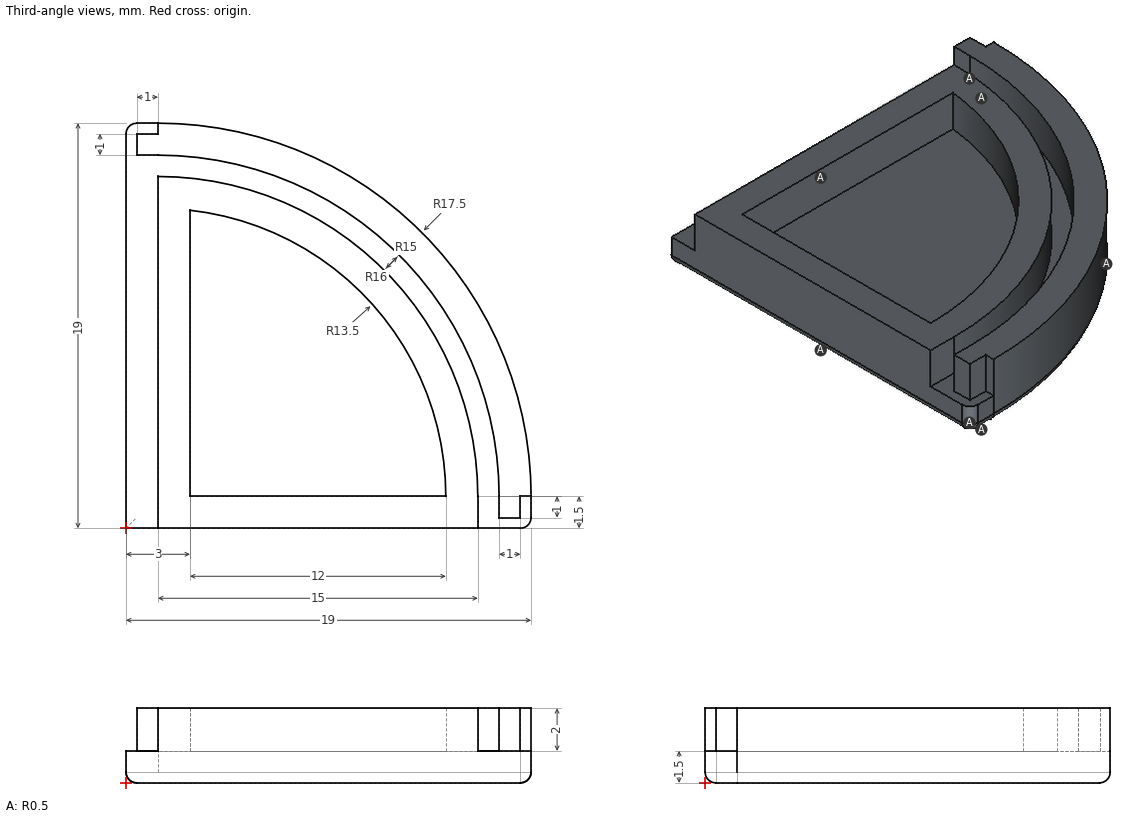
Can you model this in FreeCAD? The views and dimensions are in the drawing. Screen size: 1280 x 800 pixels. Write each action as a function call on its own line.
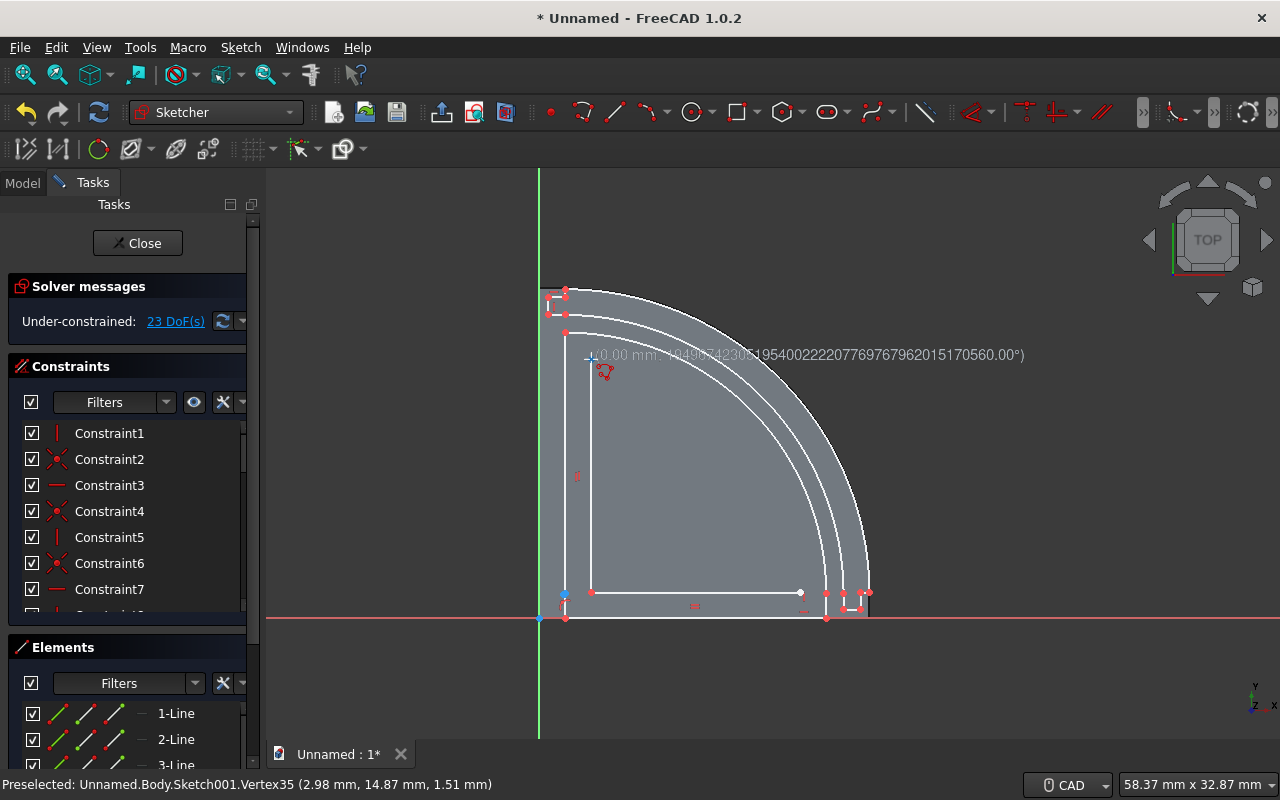
click(648, 112)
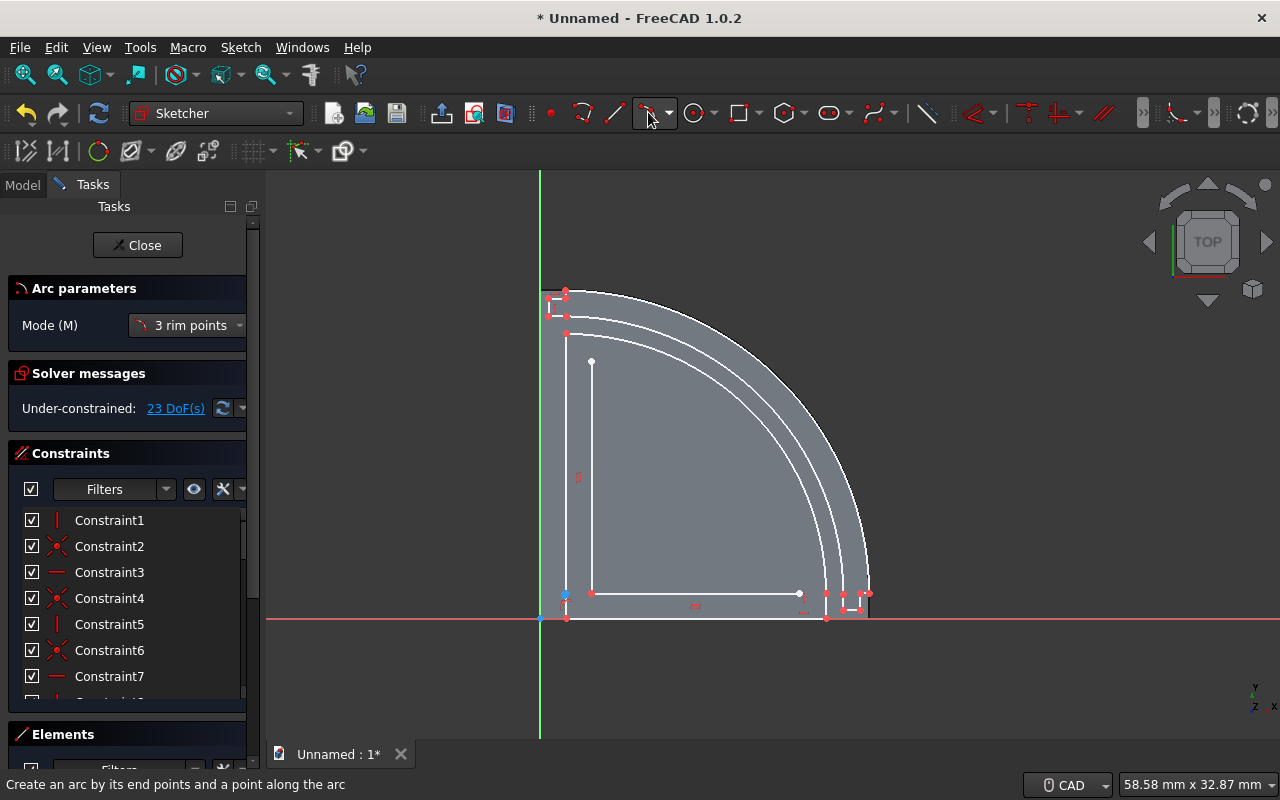
click(592, 361)
click(800, 594)
click(740, 437)
key(Escape)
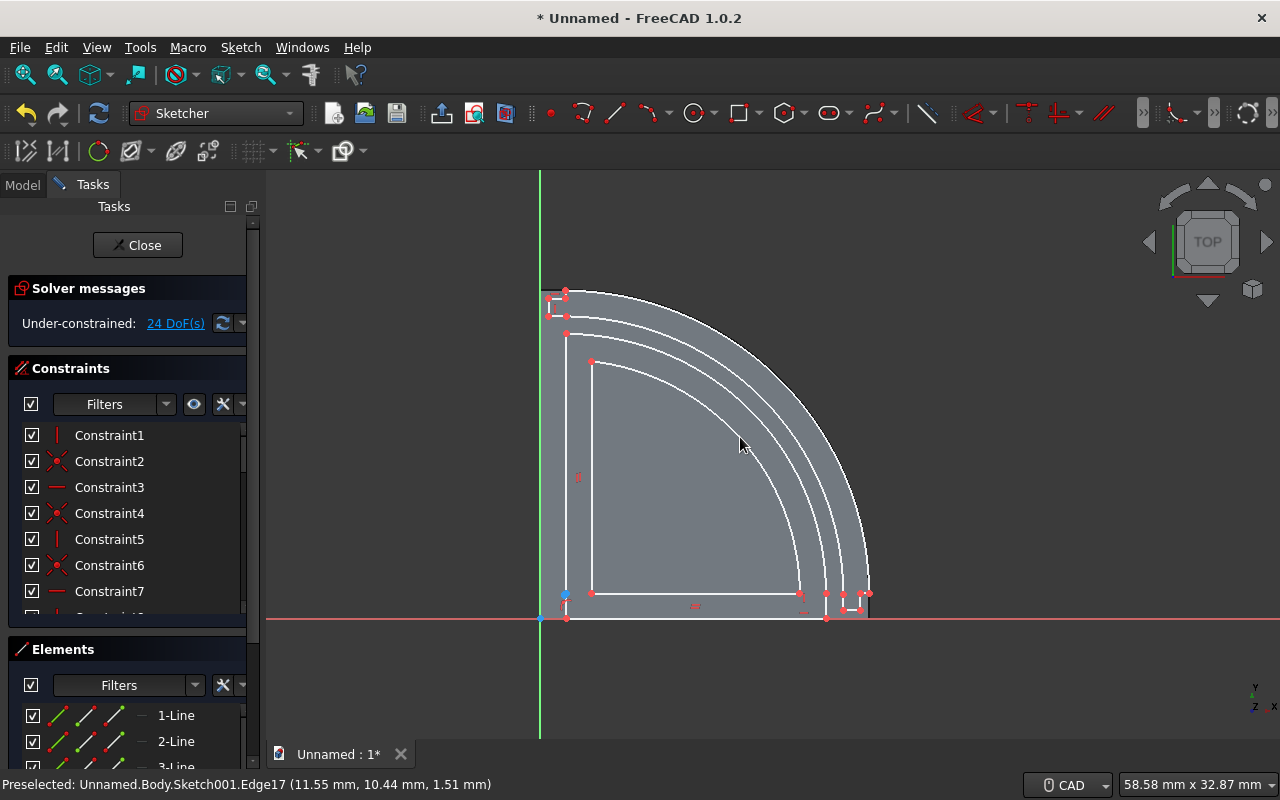
scroll(558, 316, up, 3)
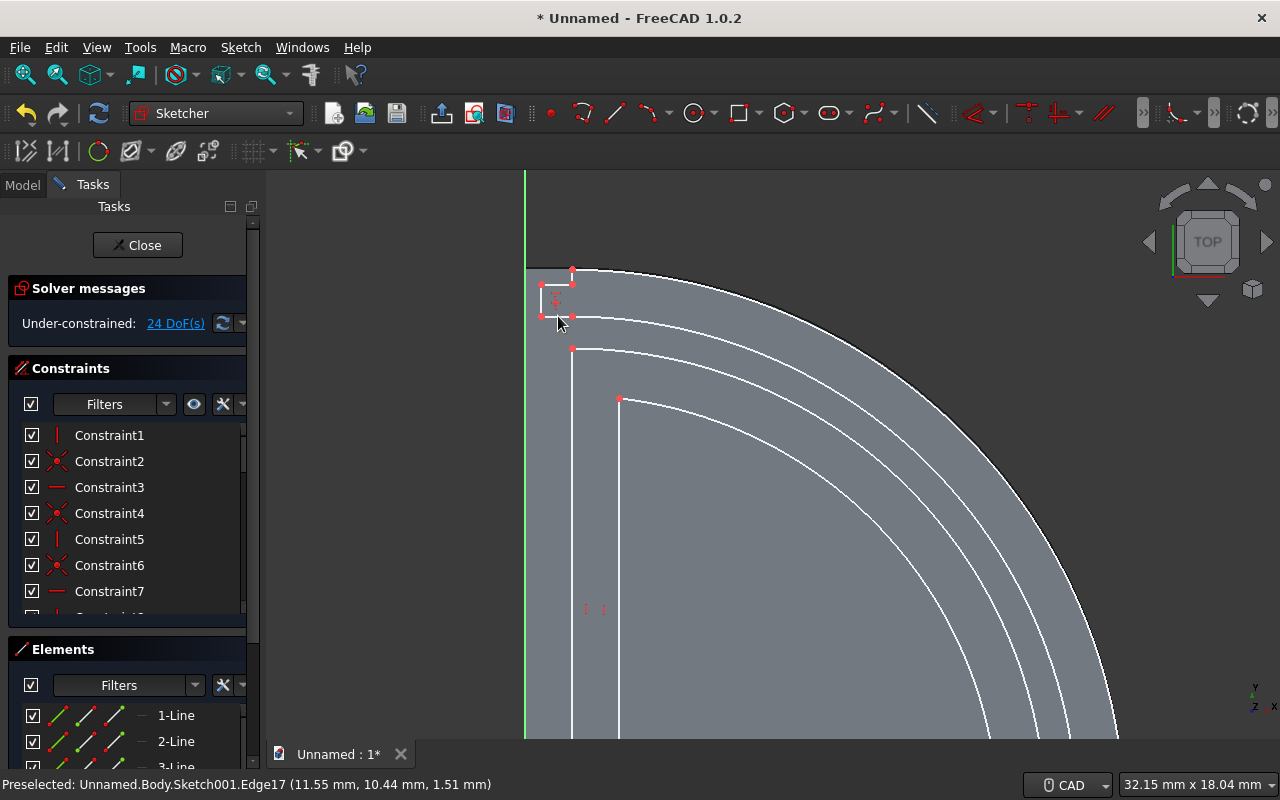
click(557, 317)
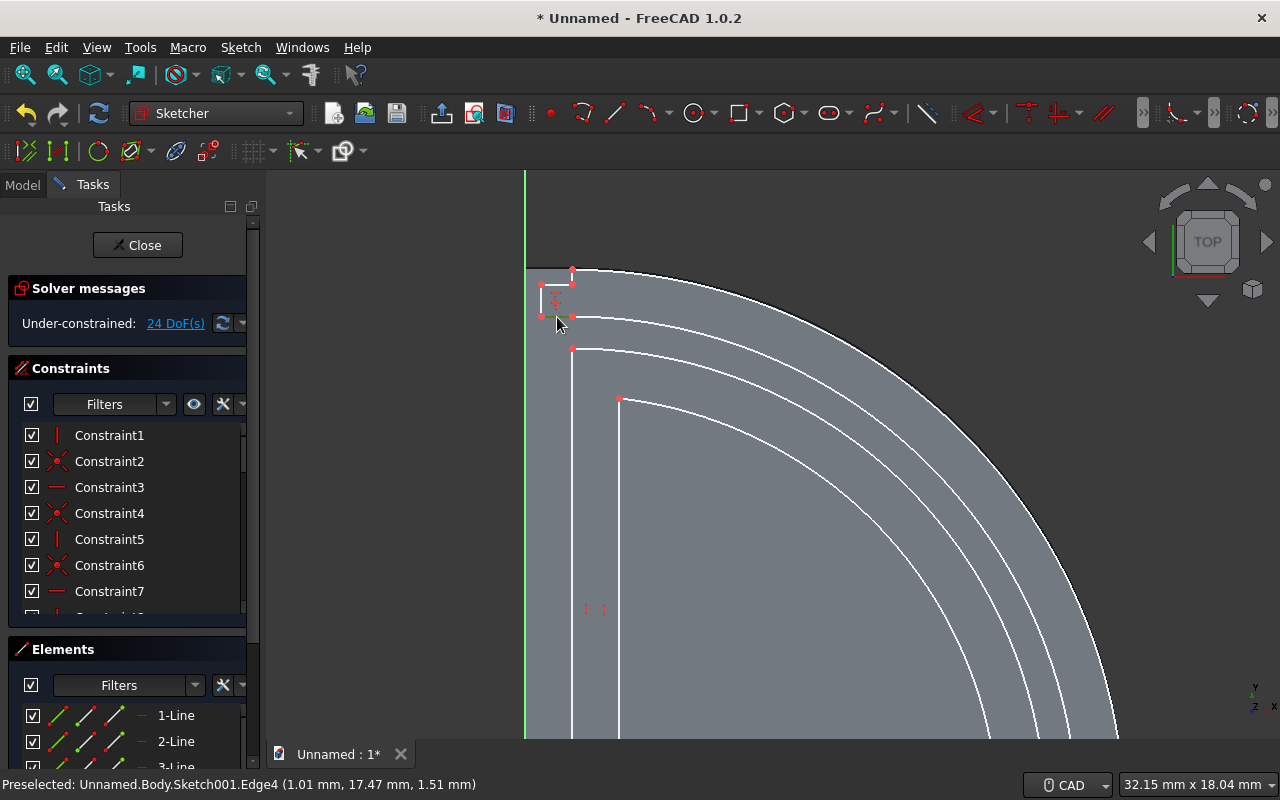
click(1022, 593)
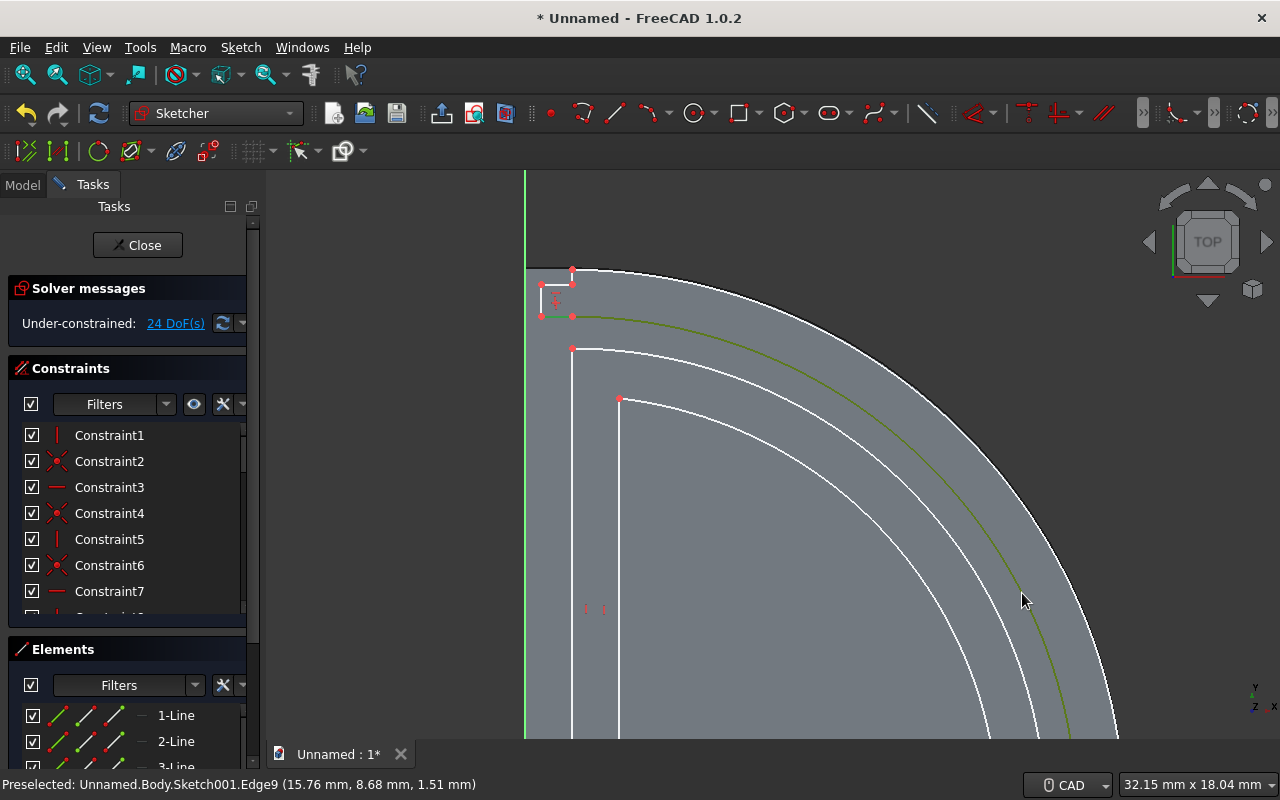
key(t)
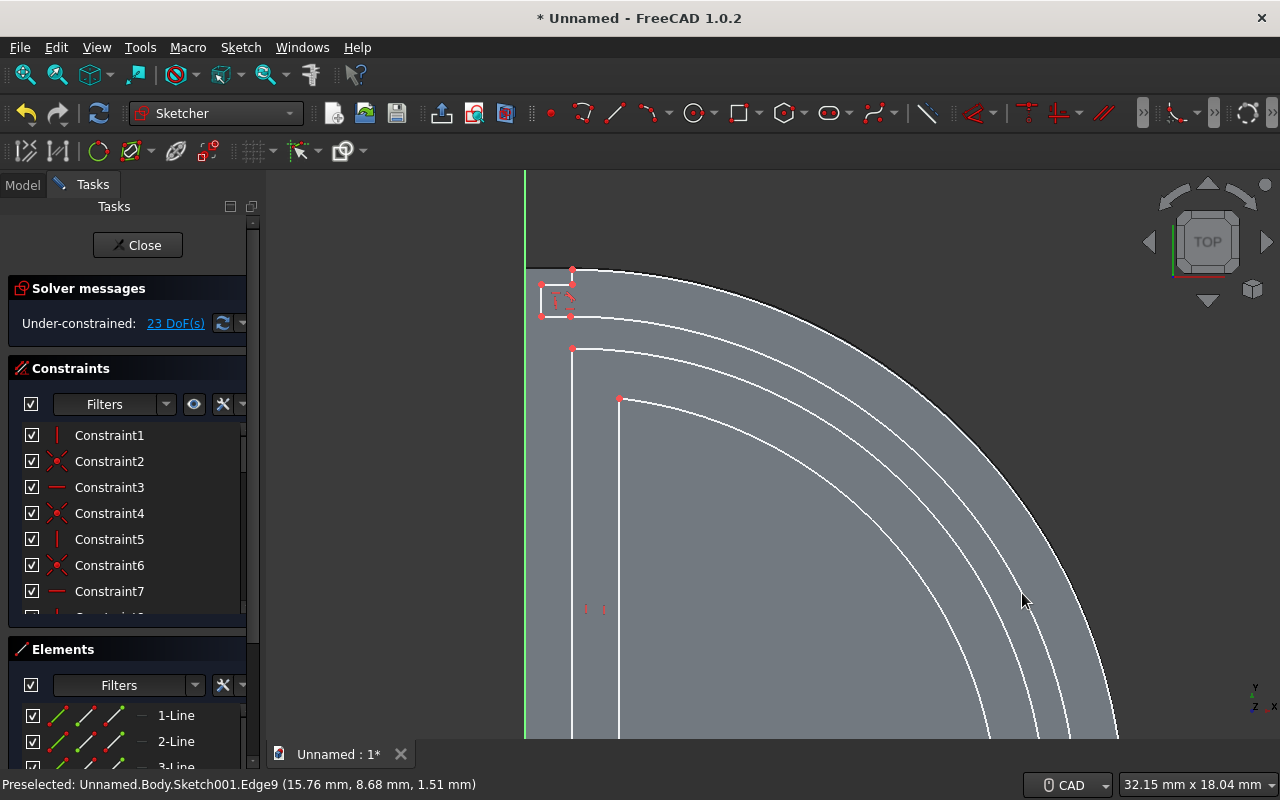
scroll(558, 317, down, 3)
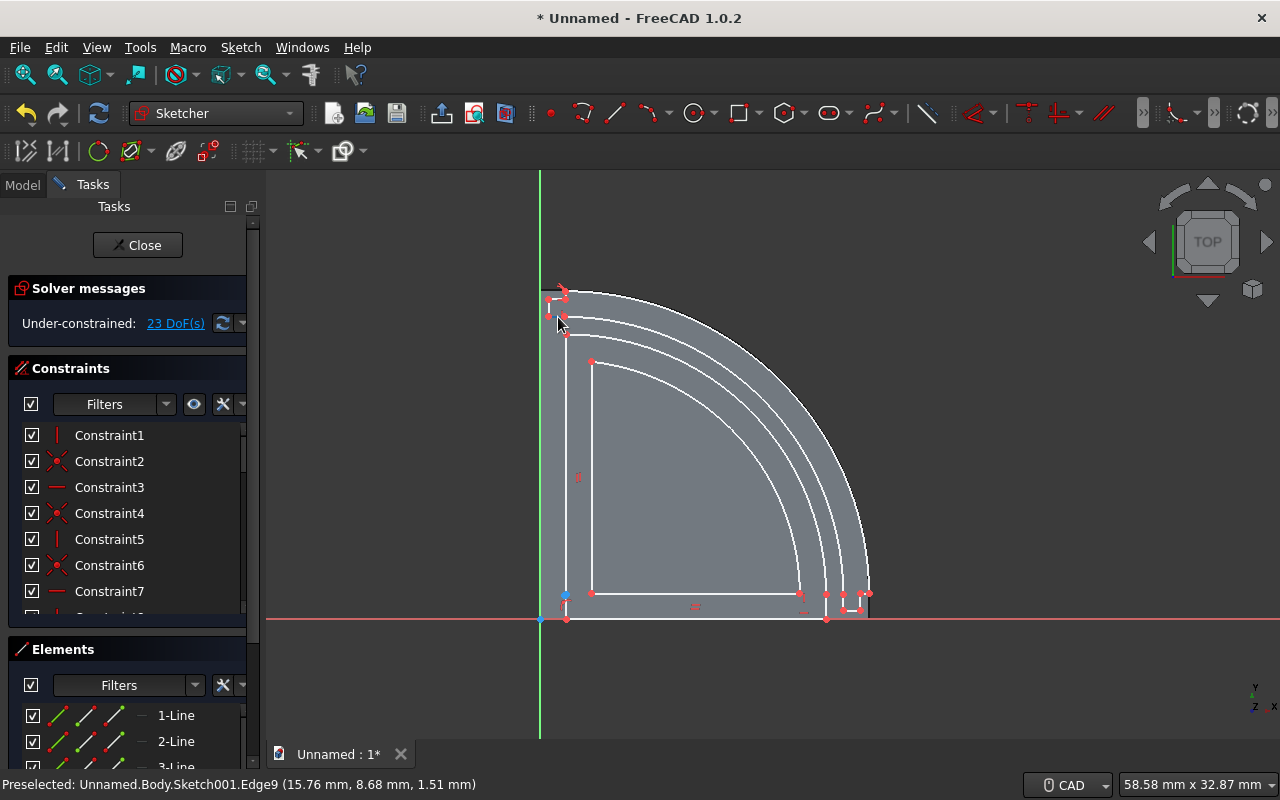
scroll(843, 601, up, 4)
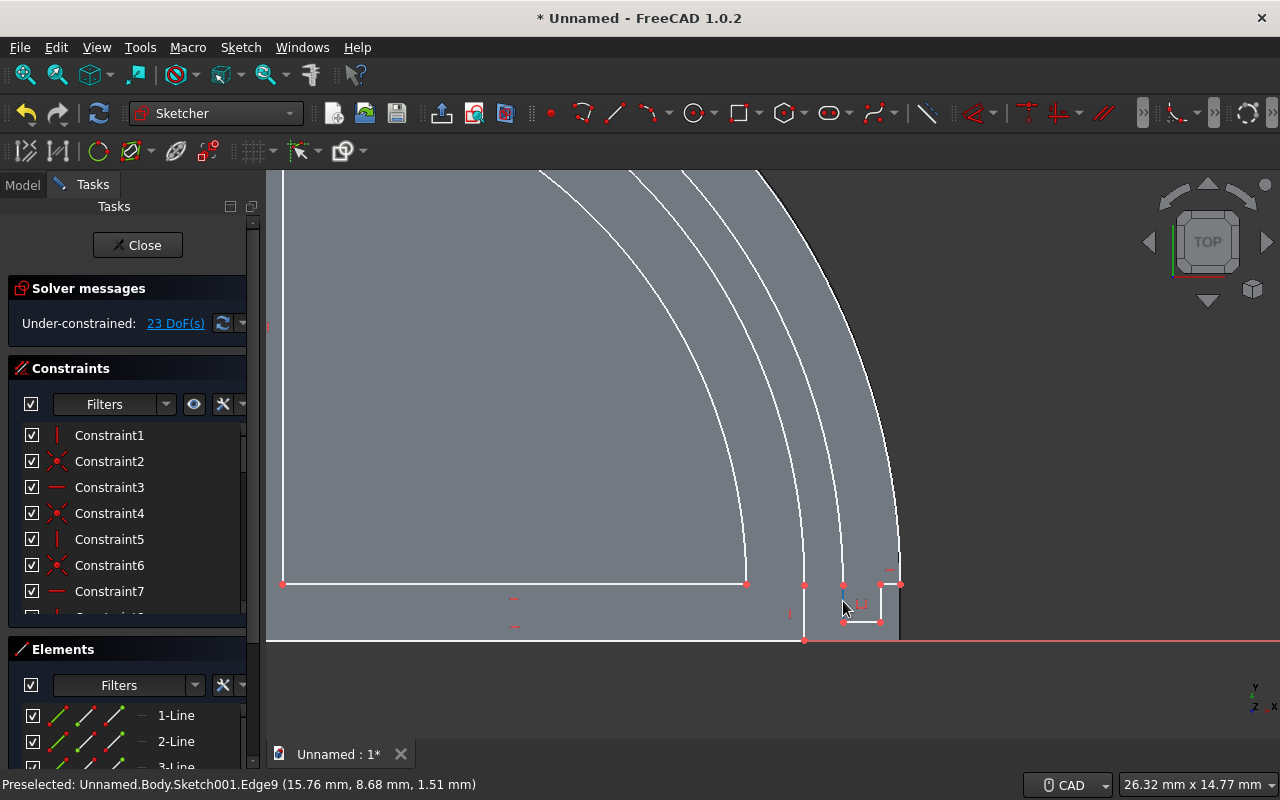
click(843, 600)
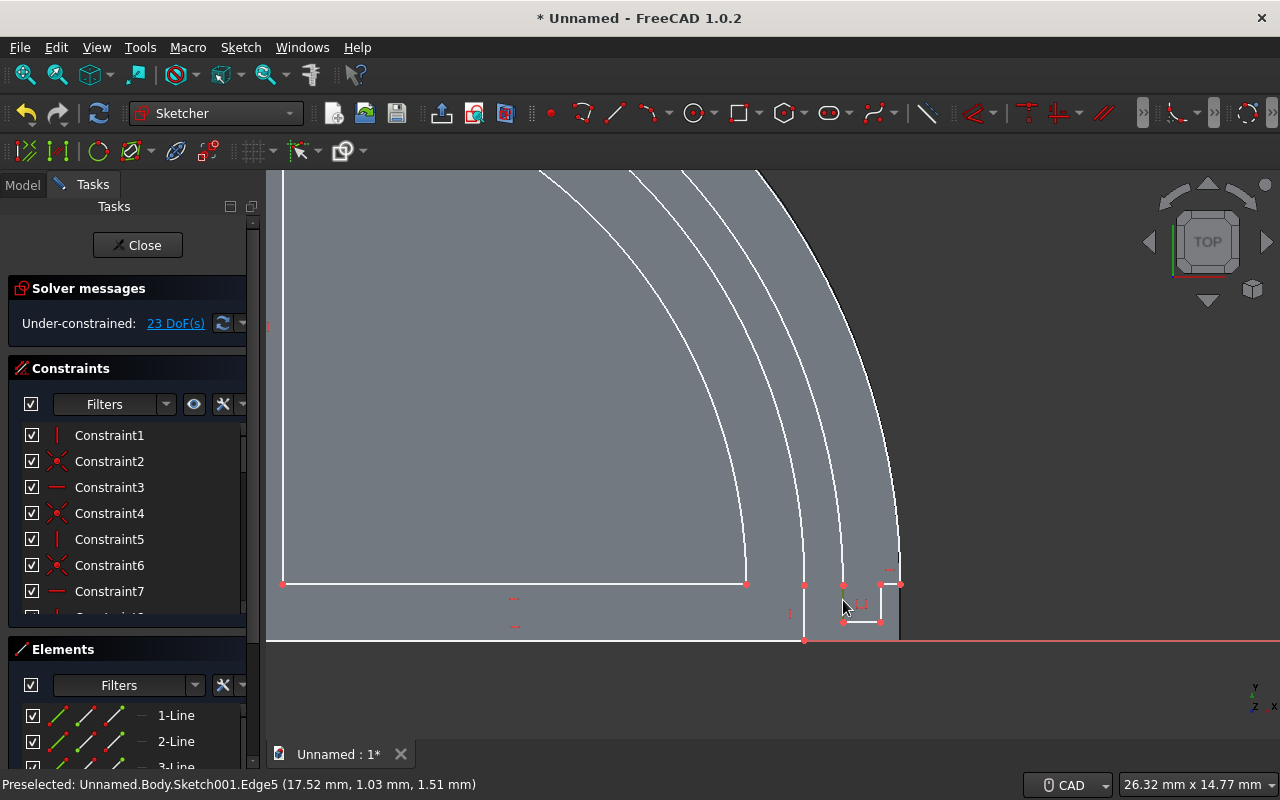
click(775, 305)